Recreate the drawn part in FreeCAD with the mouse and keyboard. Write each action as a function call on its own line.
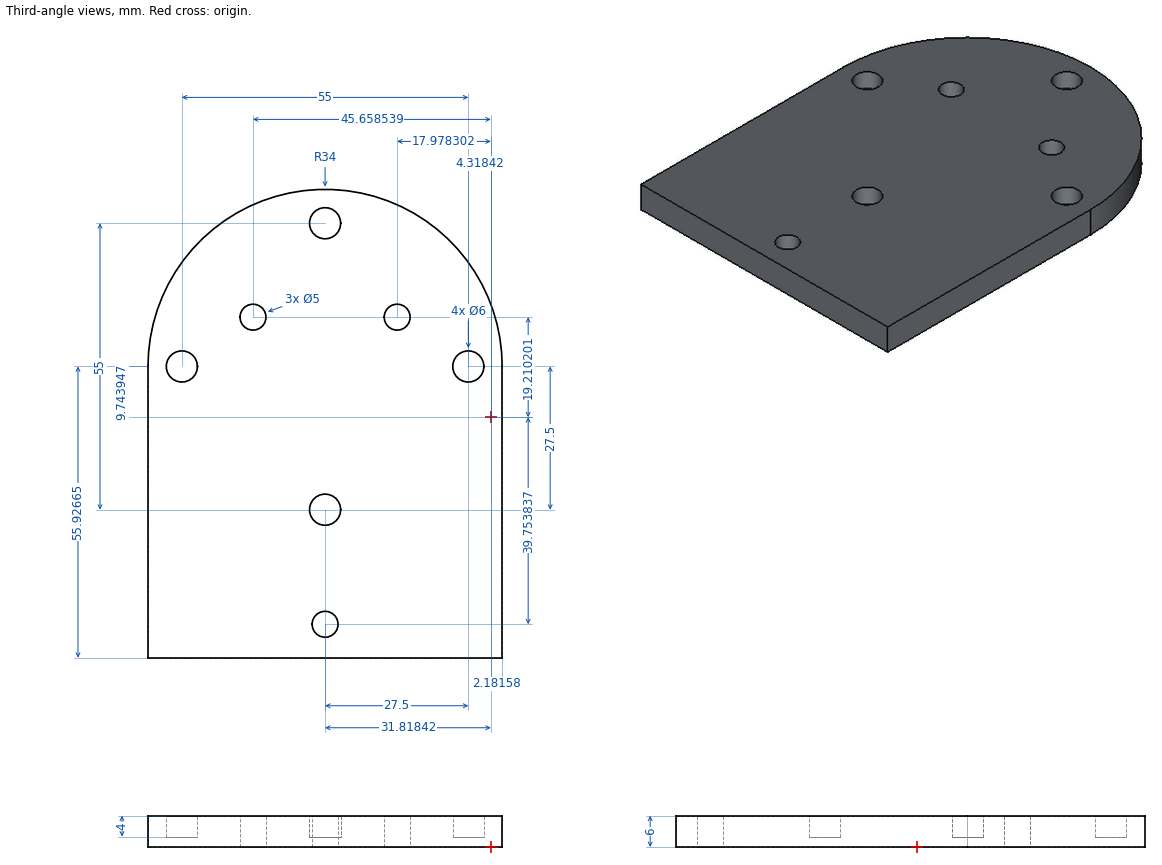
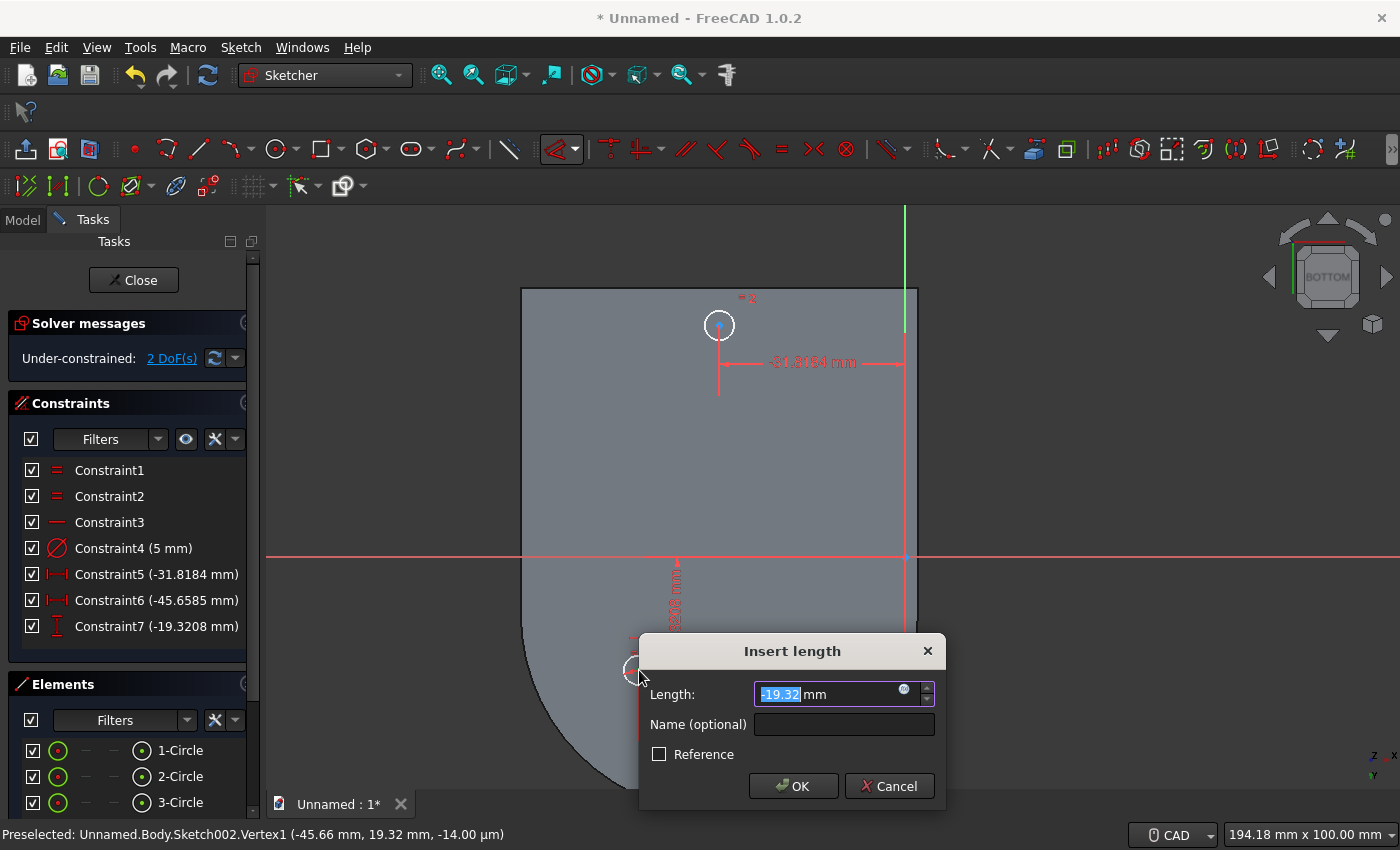
text(-19.210201)
key(Return)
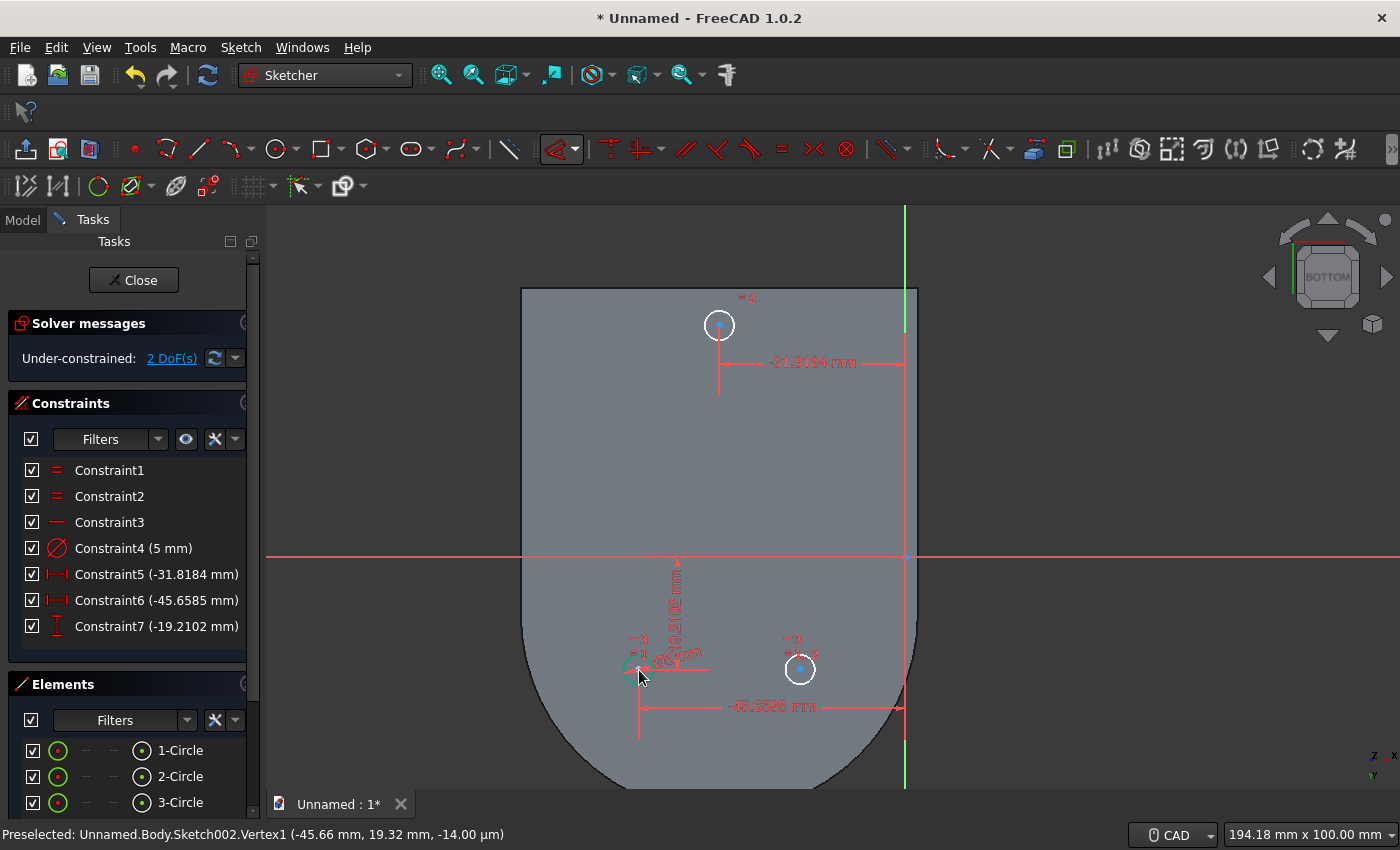
click(800, 670)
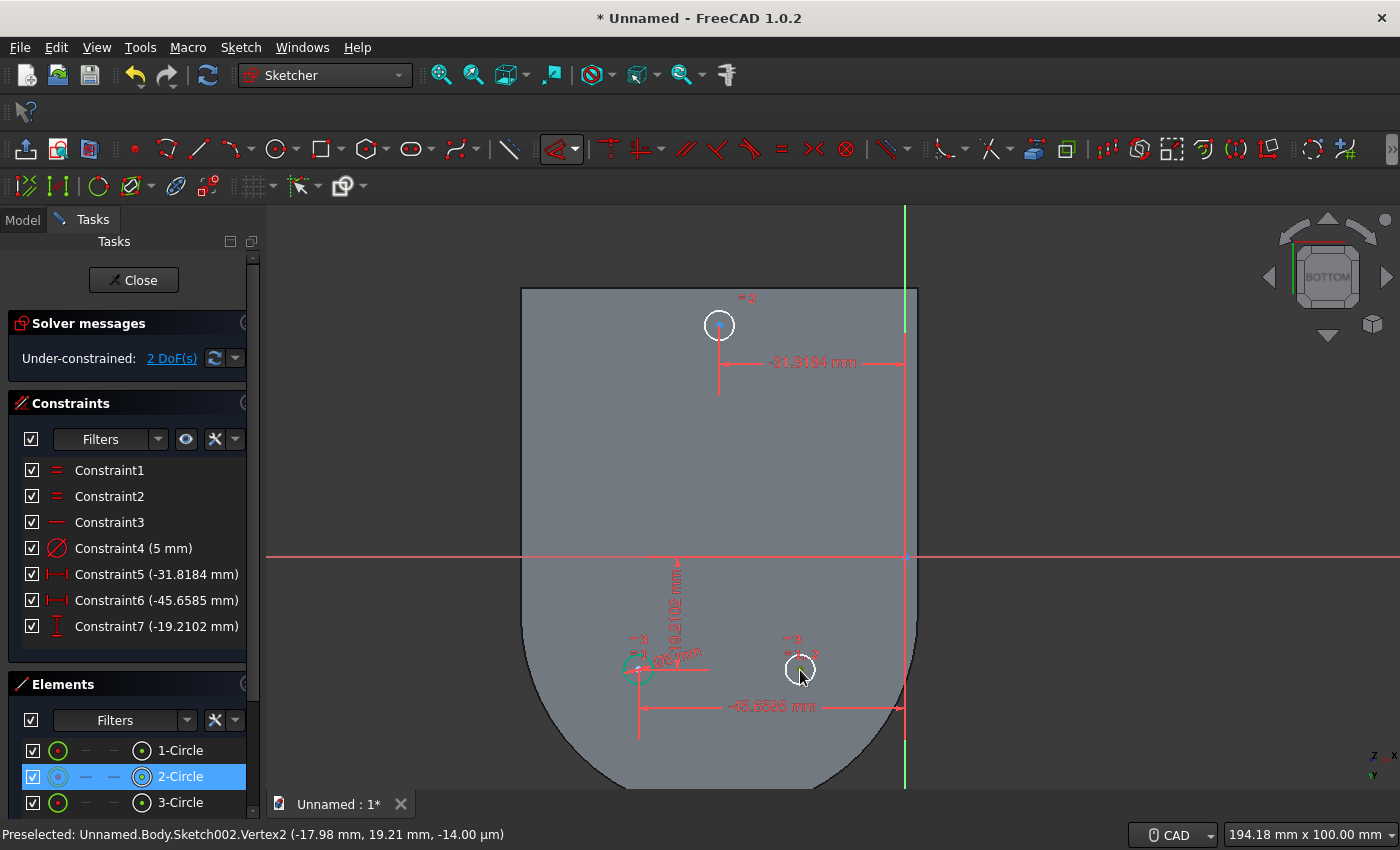
click(578, 150)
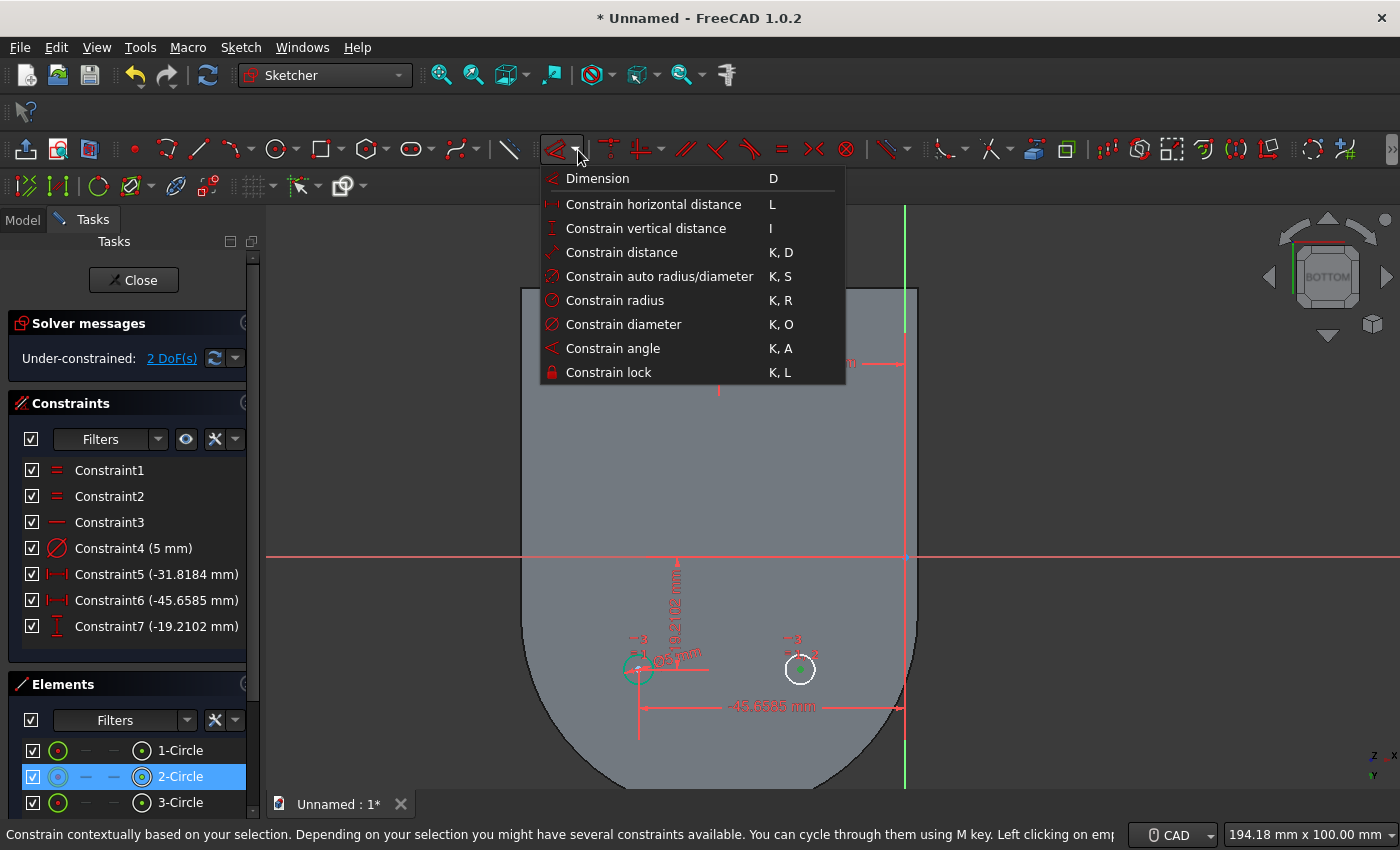
click(693, 204)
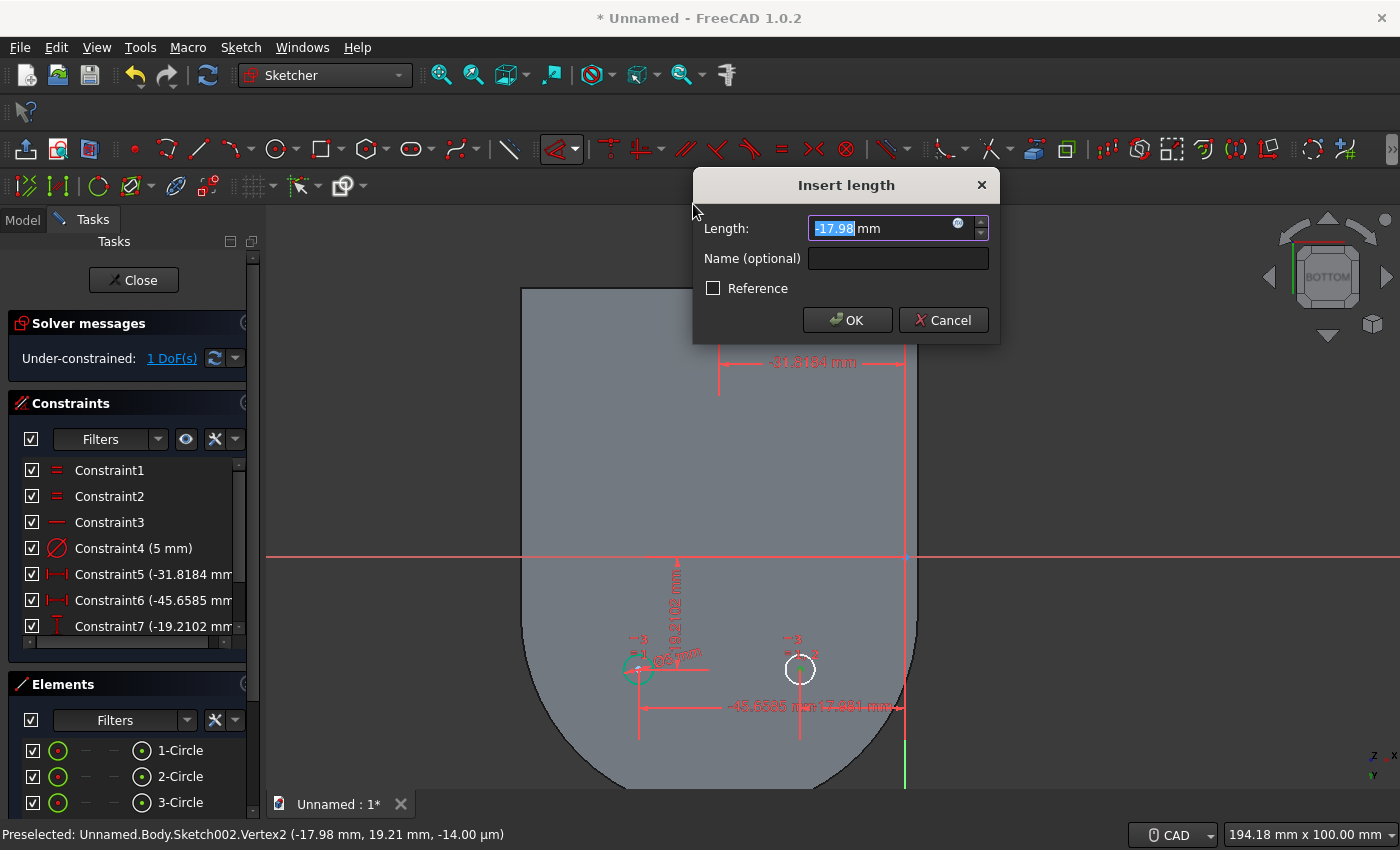
text(-17.978302)
key(Return)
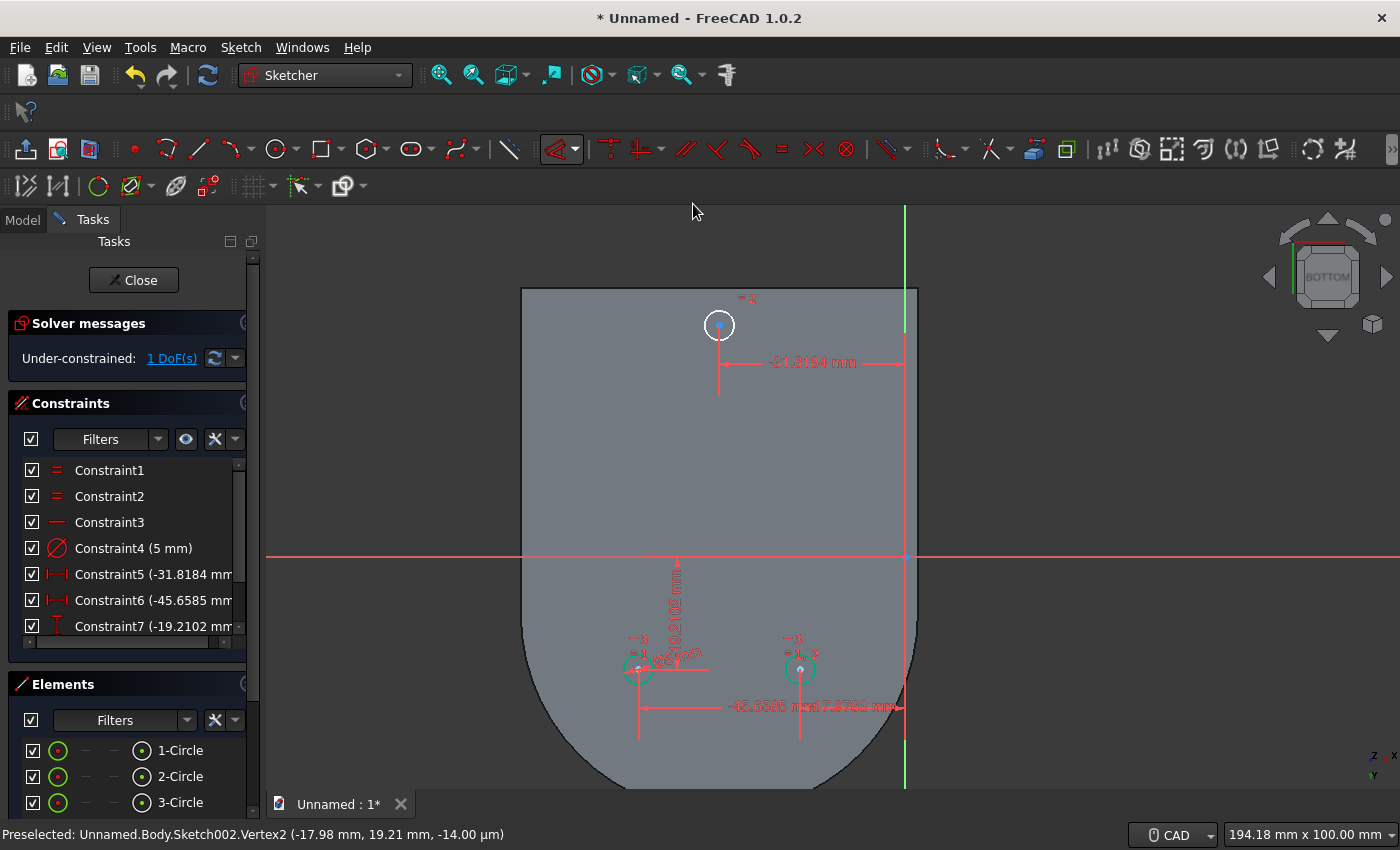
click(719, 326)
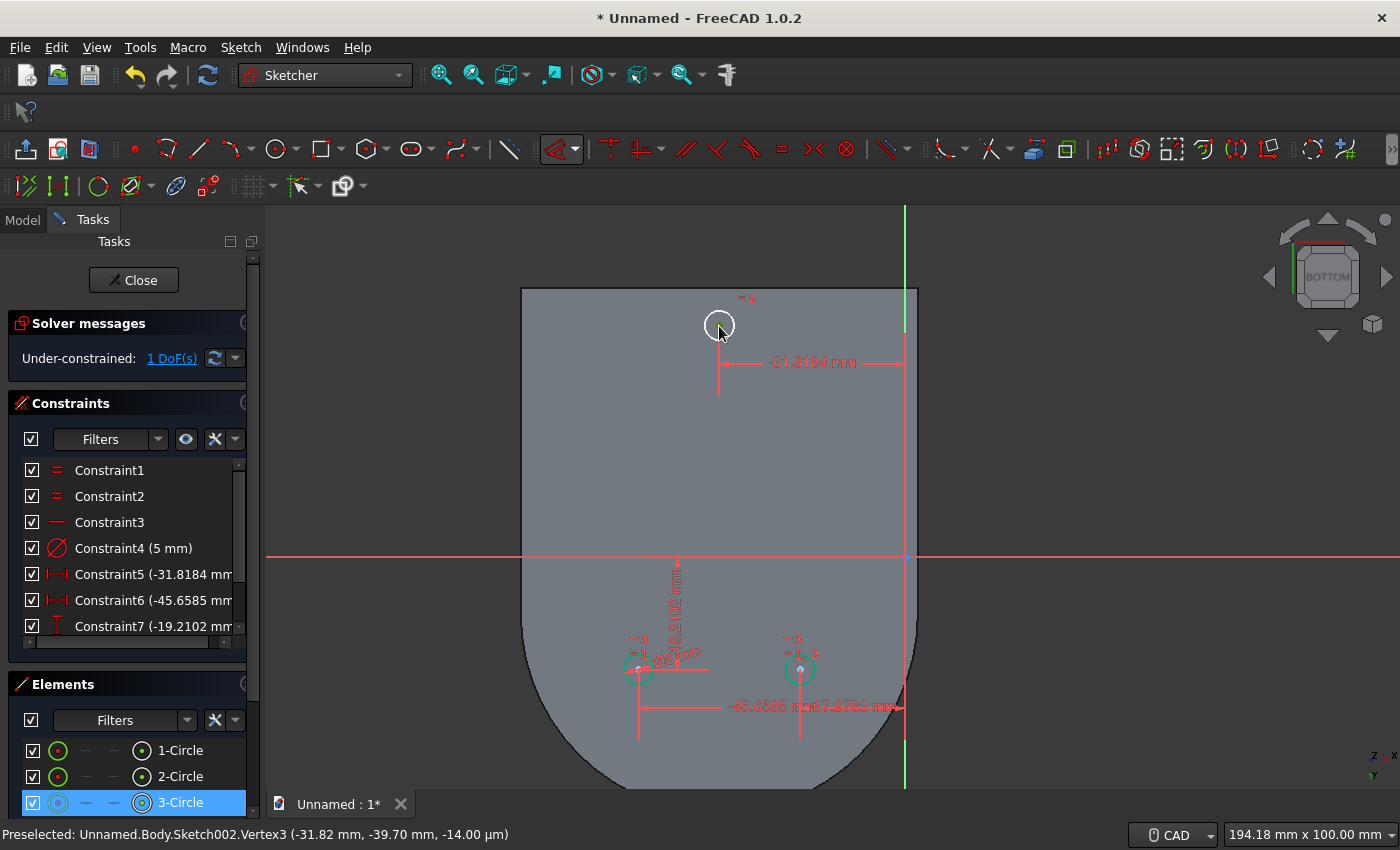
key(i)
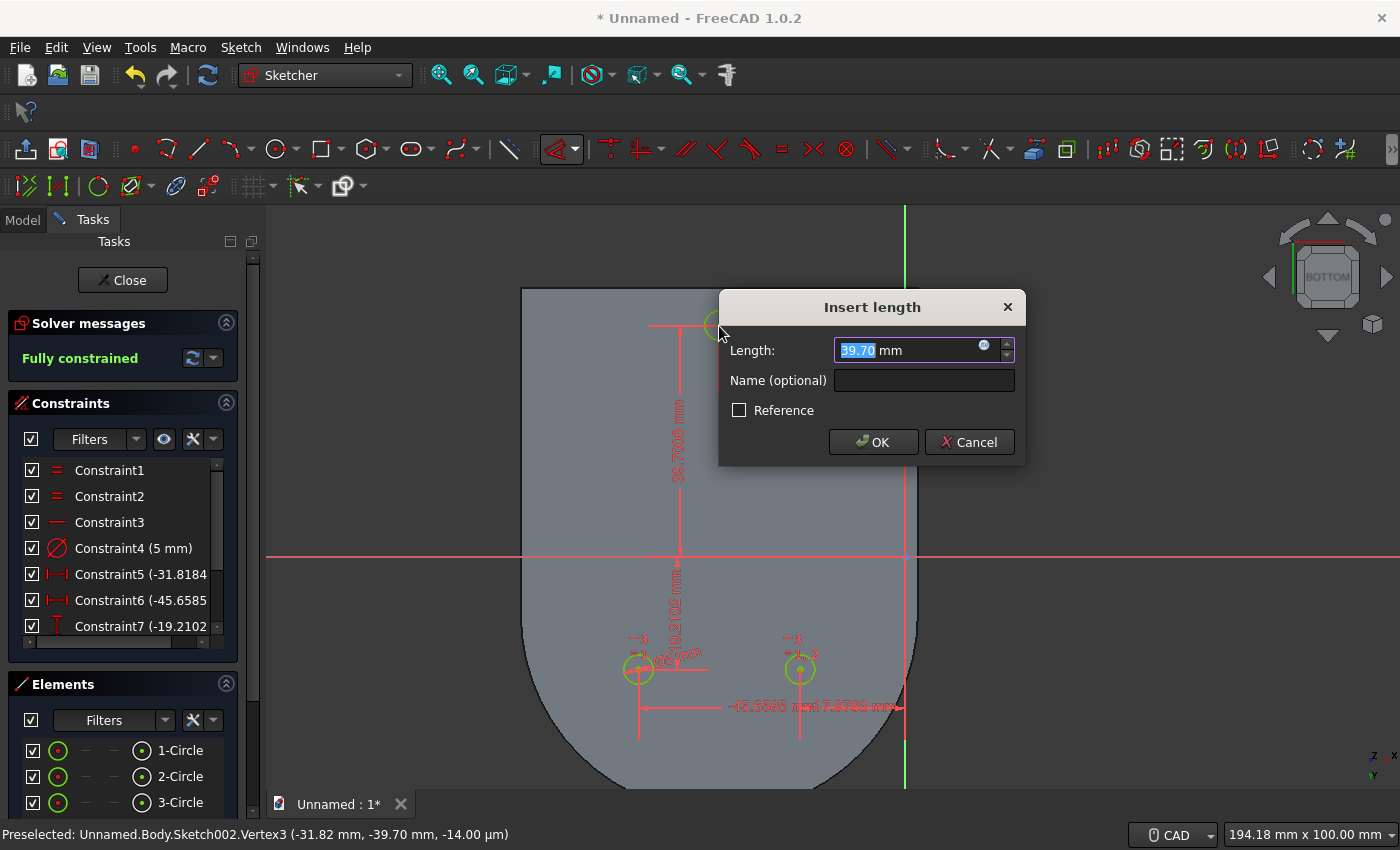
text(39.753837)
key(Return)